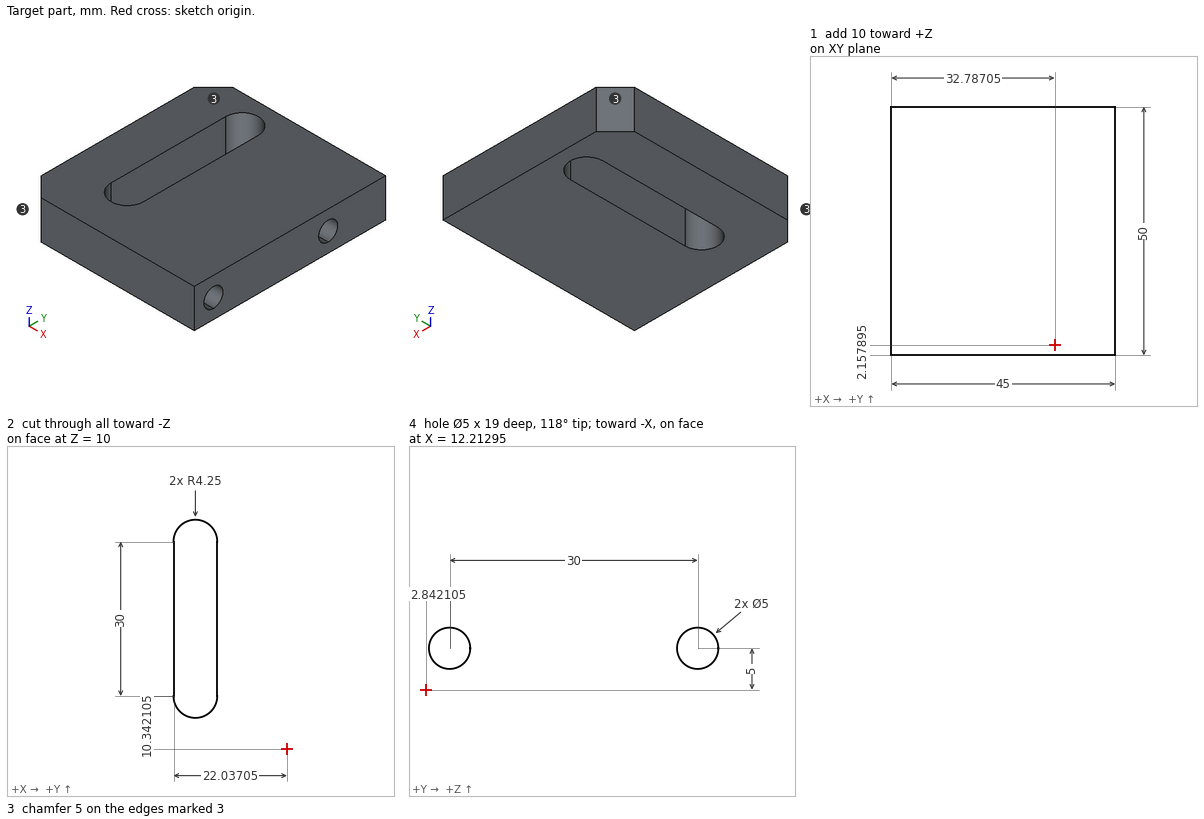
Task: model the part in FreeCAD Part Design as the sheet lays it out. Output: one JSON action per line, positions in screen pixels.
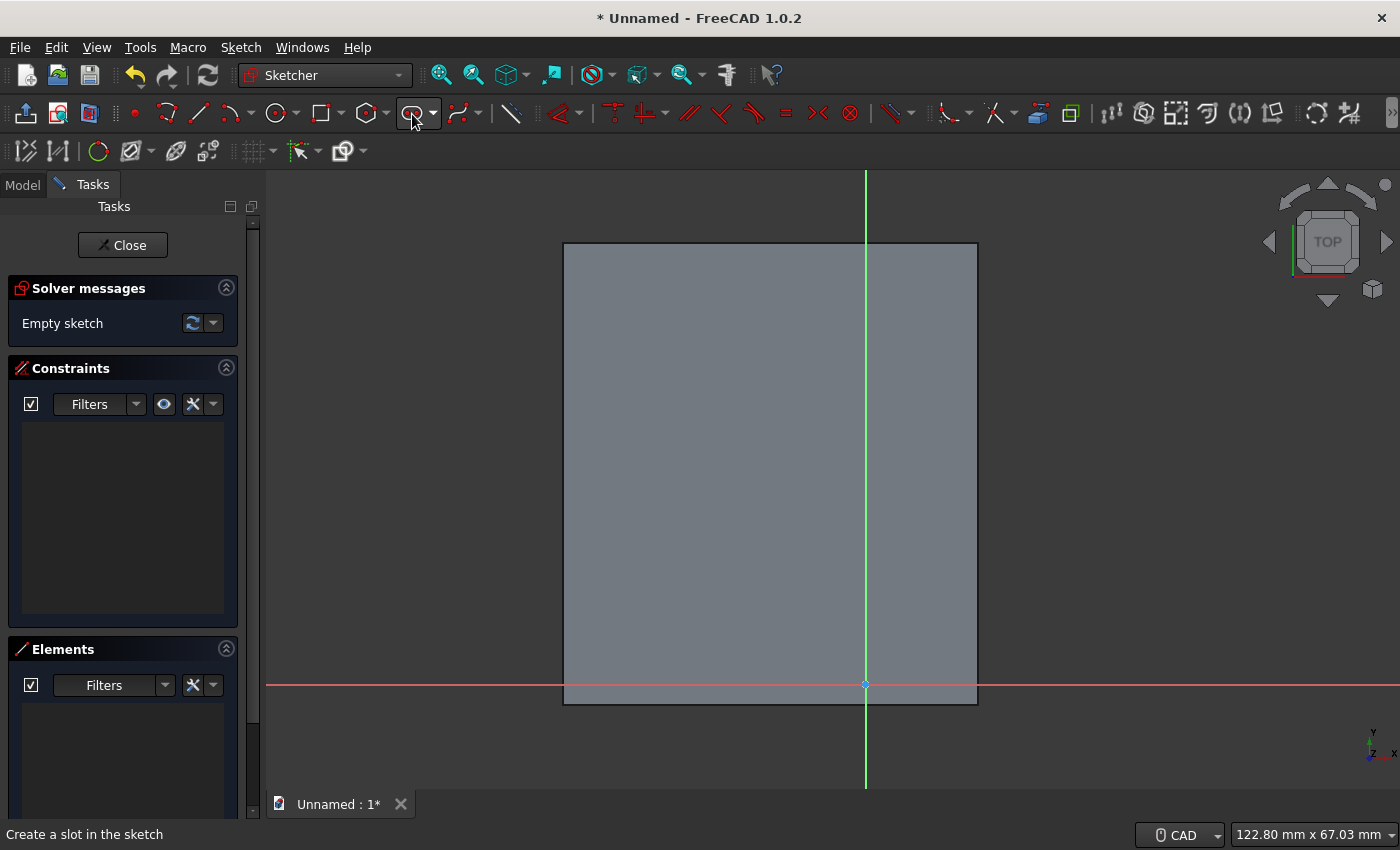
{"action": "left_click", "coordinate": [701, 589]}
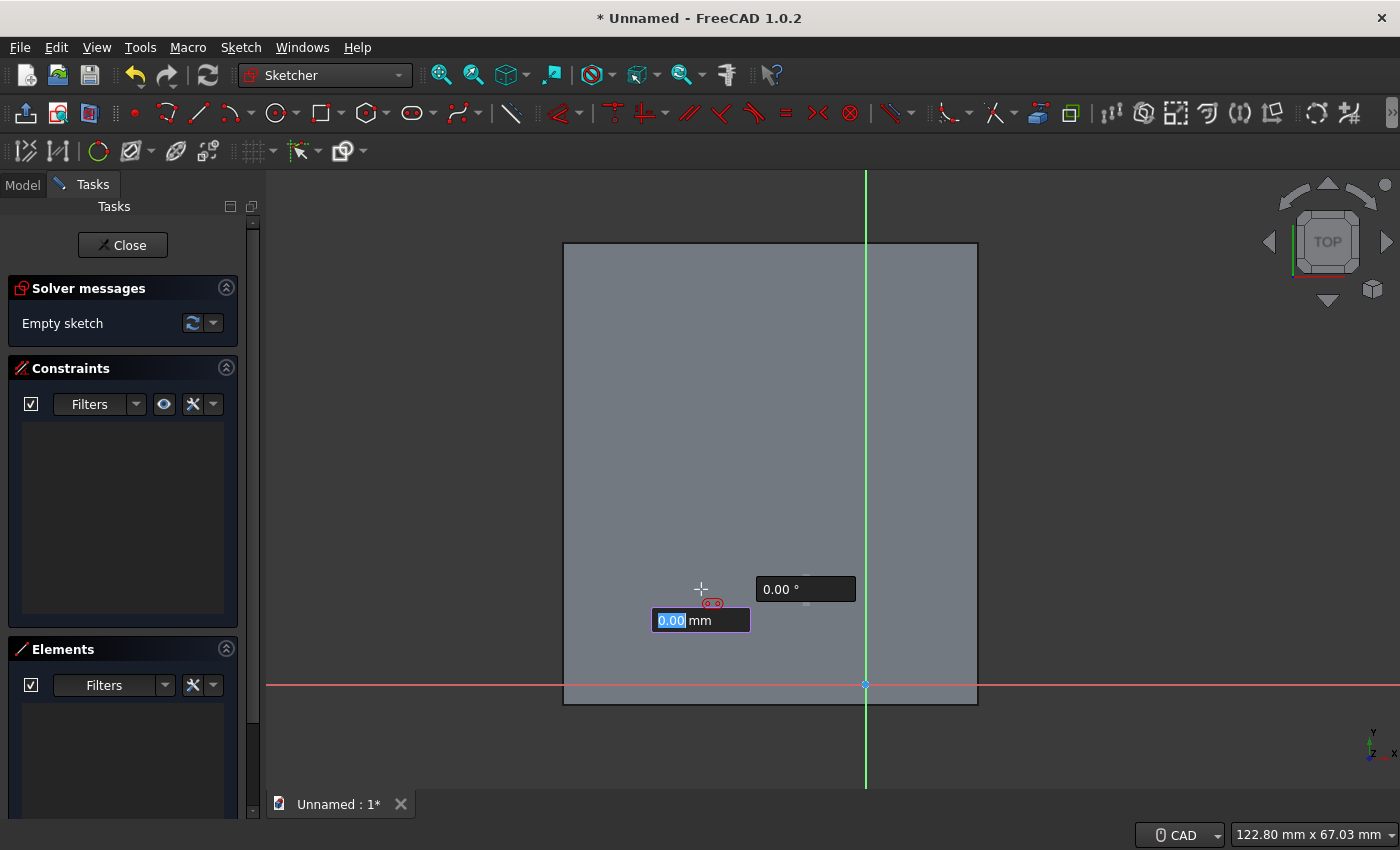
{"action": "left_click", "coordinate": [701, 312]}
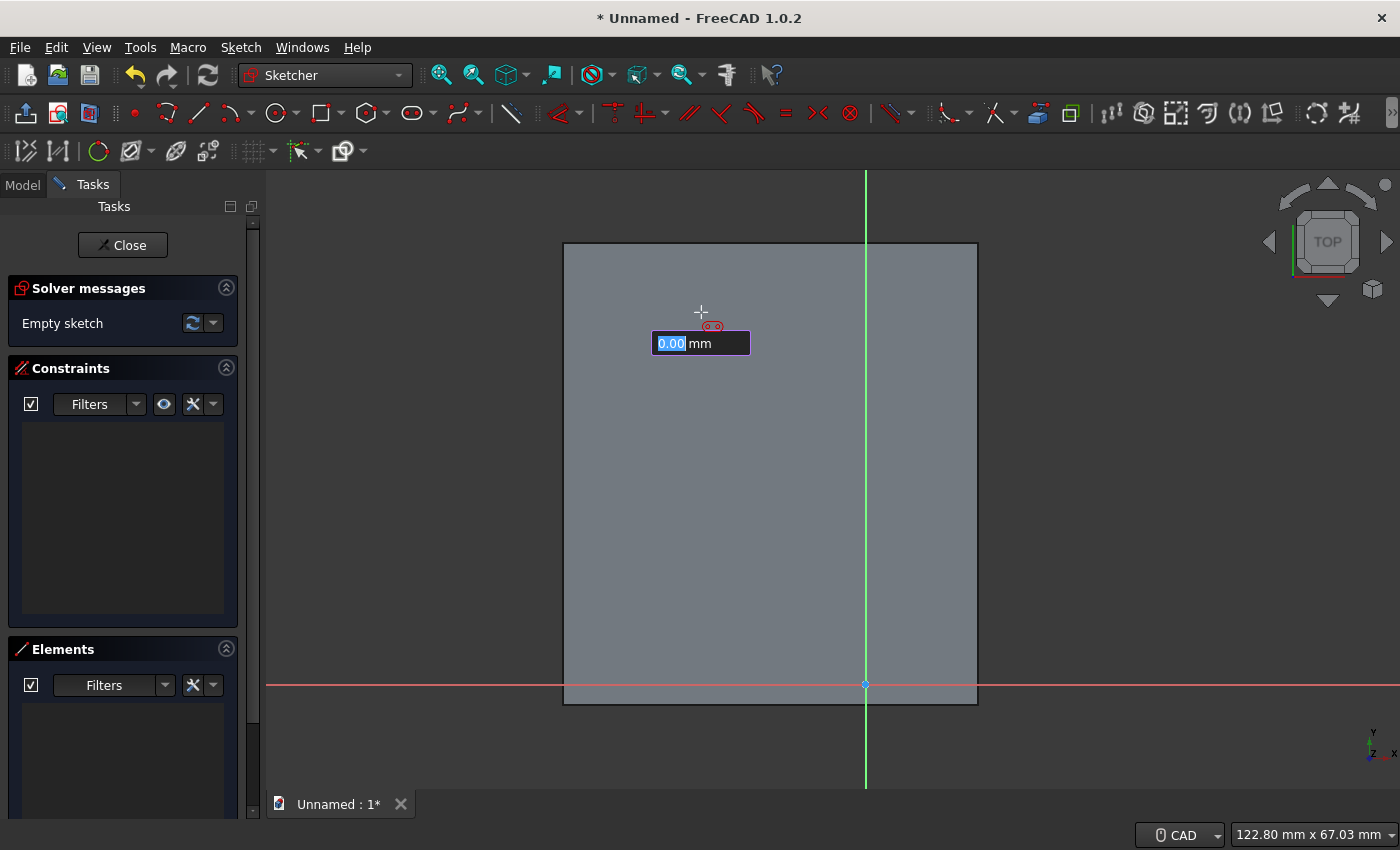
{"action": "left_click", "coordinate": [741, 451]}
{"action": "key", "text": "Escape"}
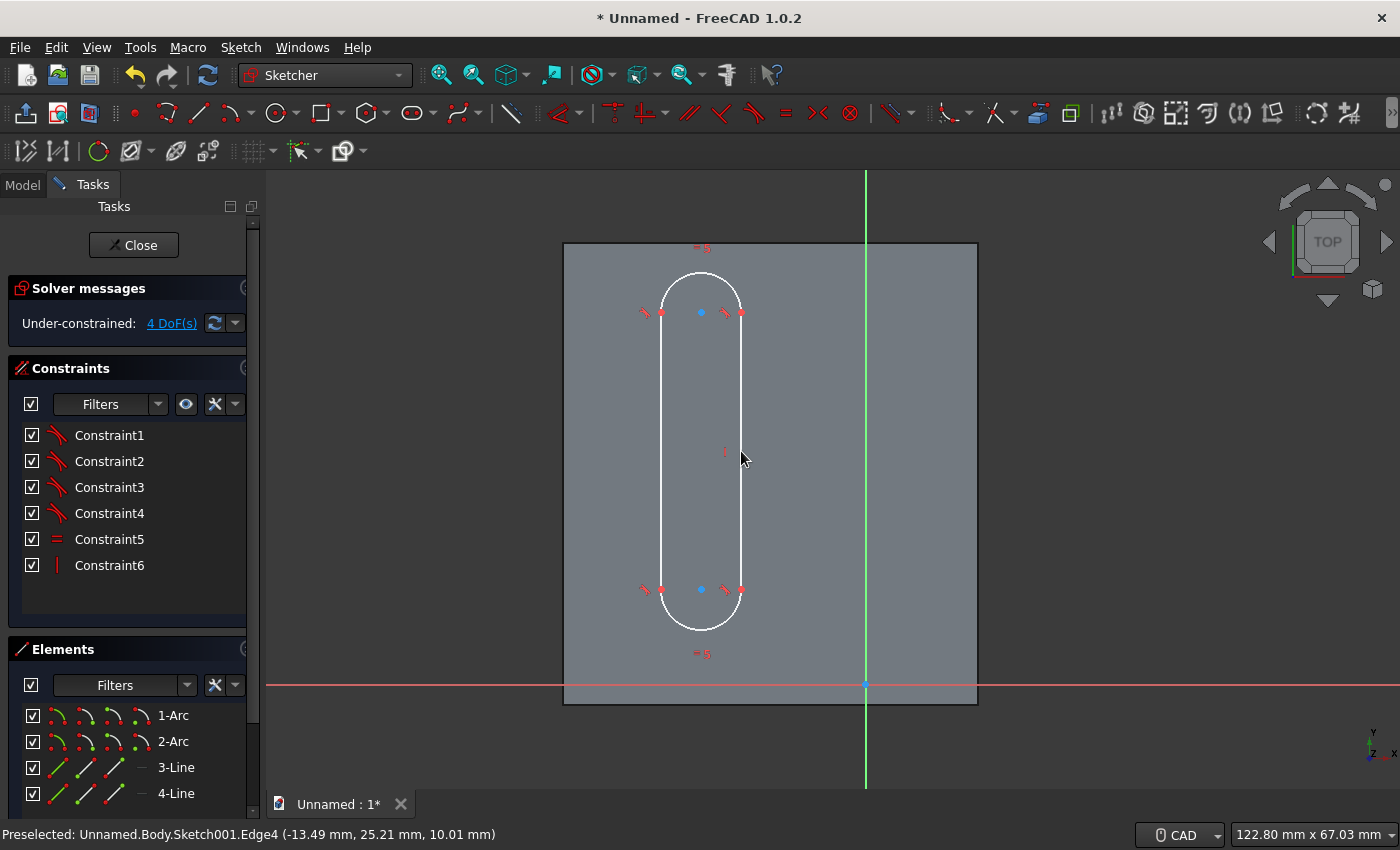
{"action": "left_click", "coordinate": [558, 114]}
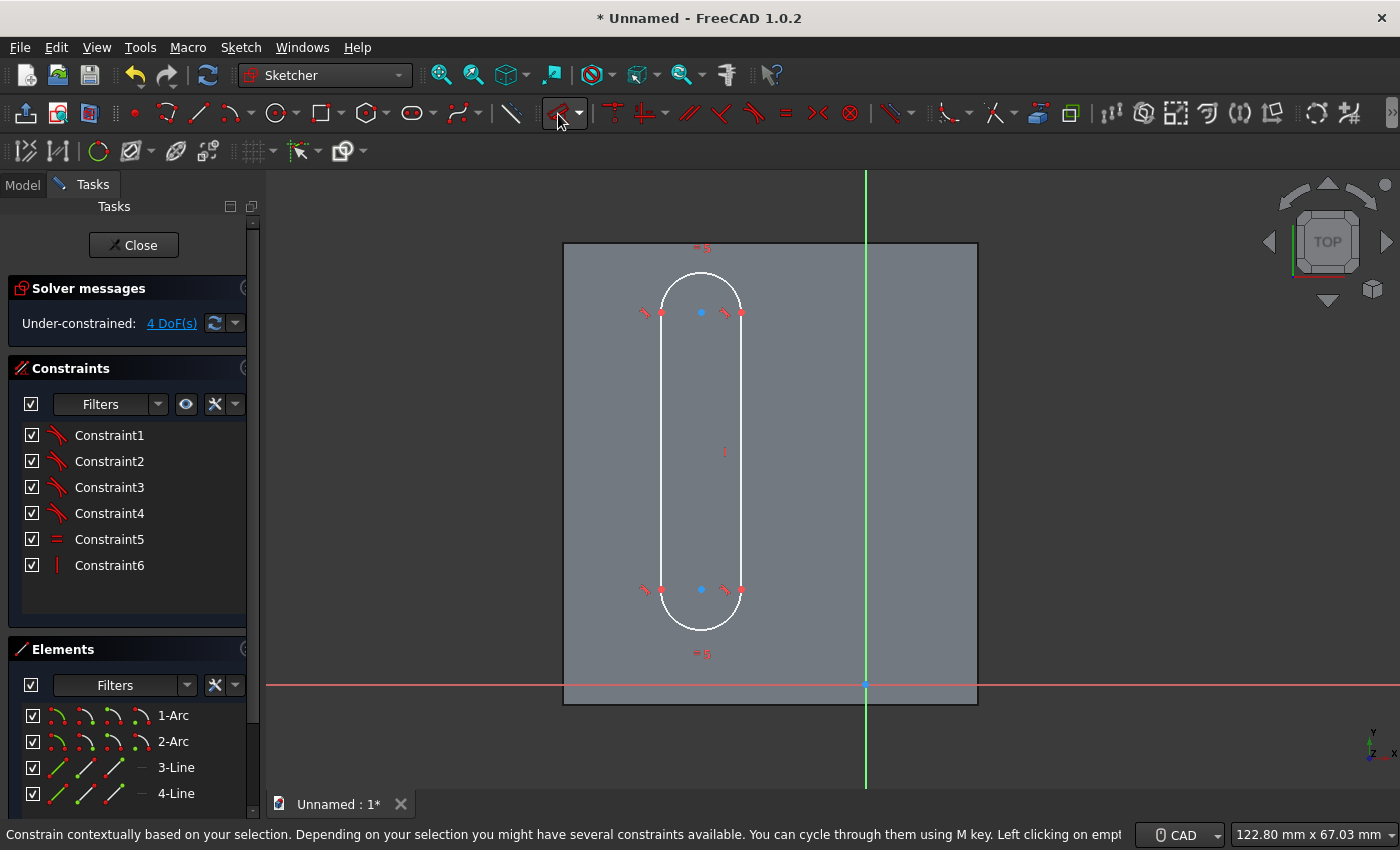
{"action": "left_click", "coordinate": [677, 622]}
{"action": "left_click", "coordinate": [658, 648]}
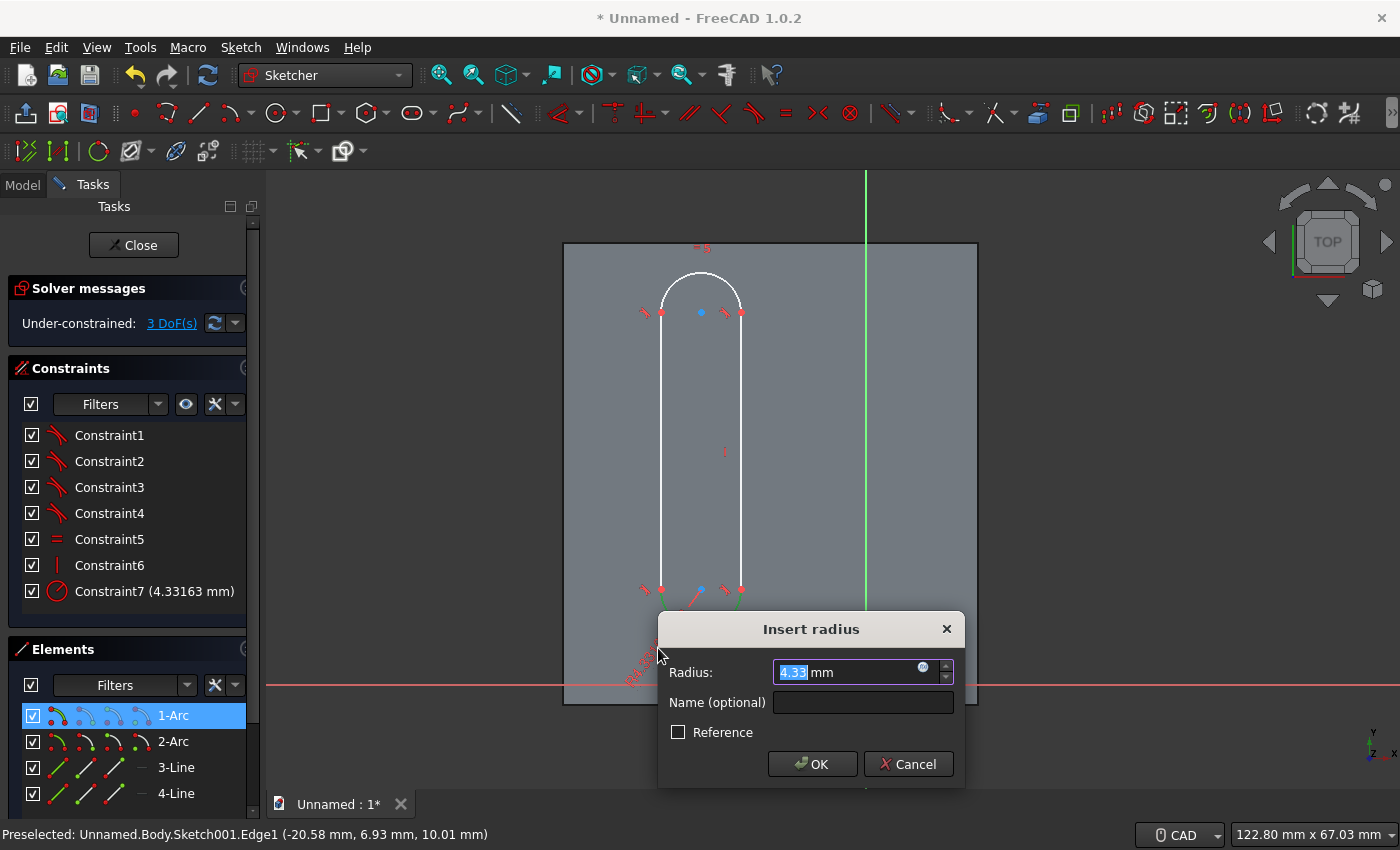
{"action": "type", "text": "4.25"}
{"action": "key", "text": "Return"}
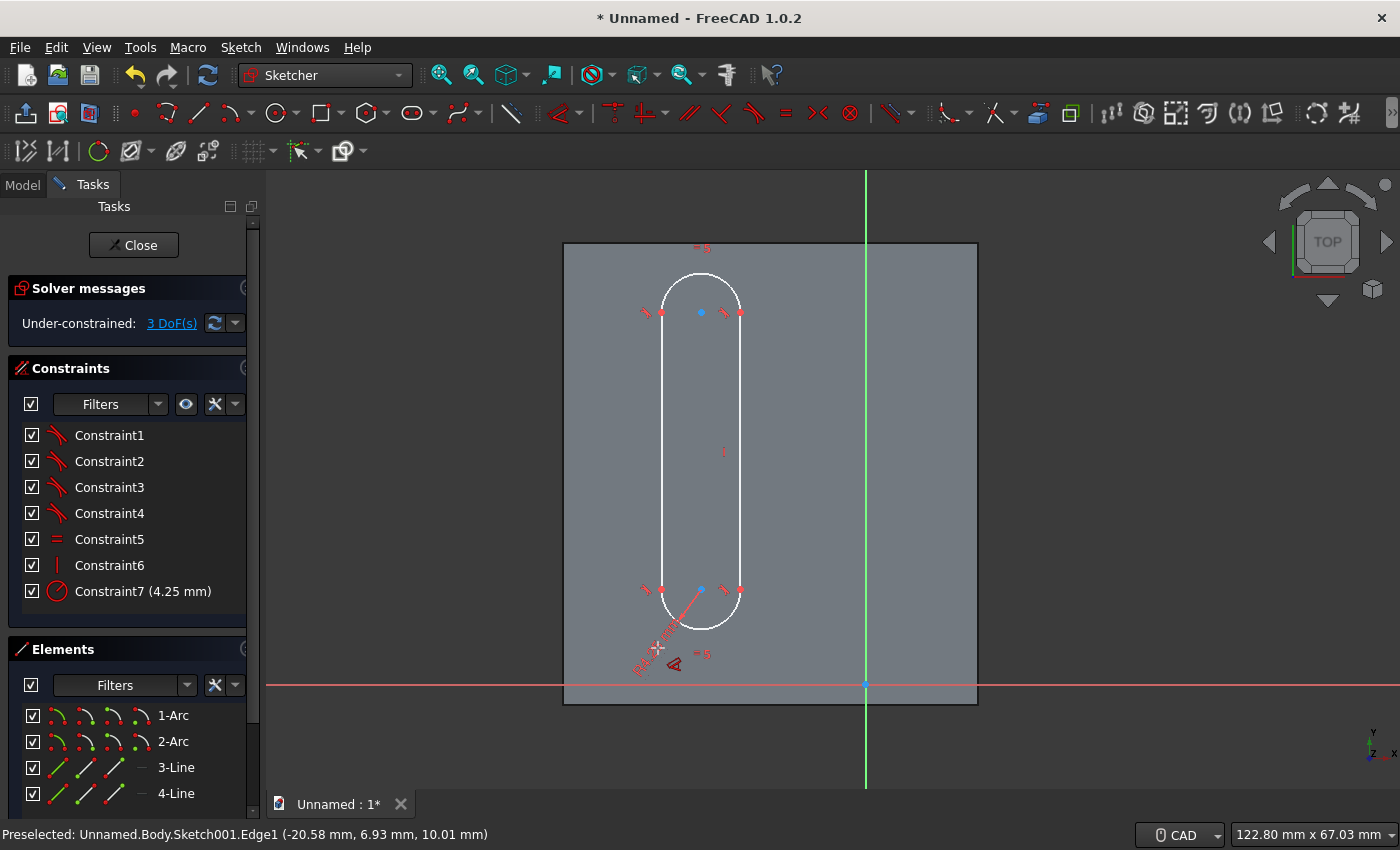
{"action": "left_click", "coordinate": [662, 507]}
{"action": "left_click", "coordinate": [628, 452]}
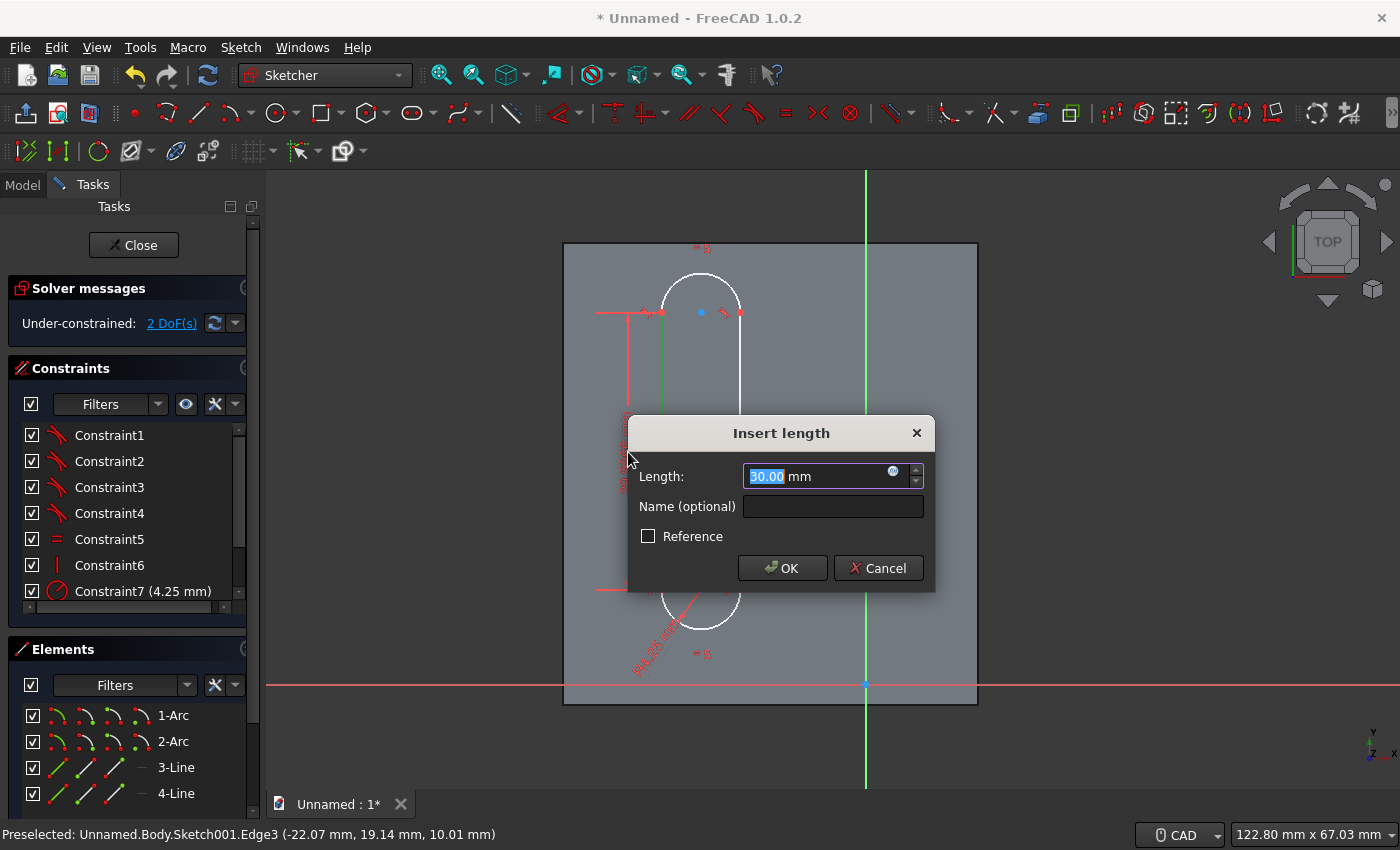
{"action": "type", "text": "30"}
{"action": "key", "text": "Return"}